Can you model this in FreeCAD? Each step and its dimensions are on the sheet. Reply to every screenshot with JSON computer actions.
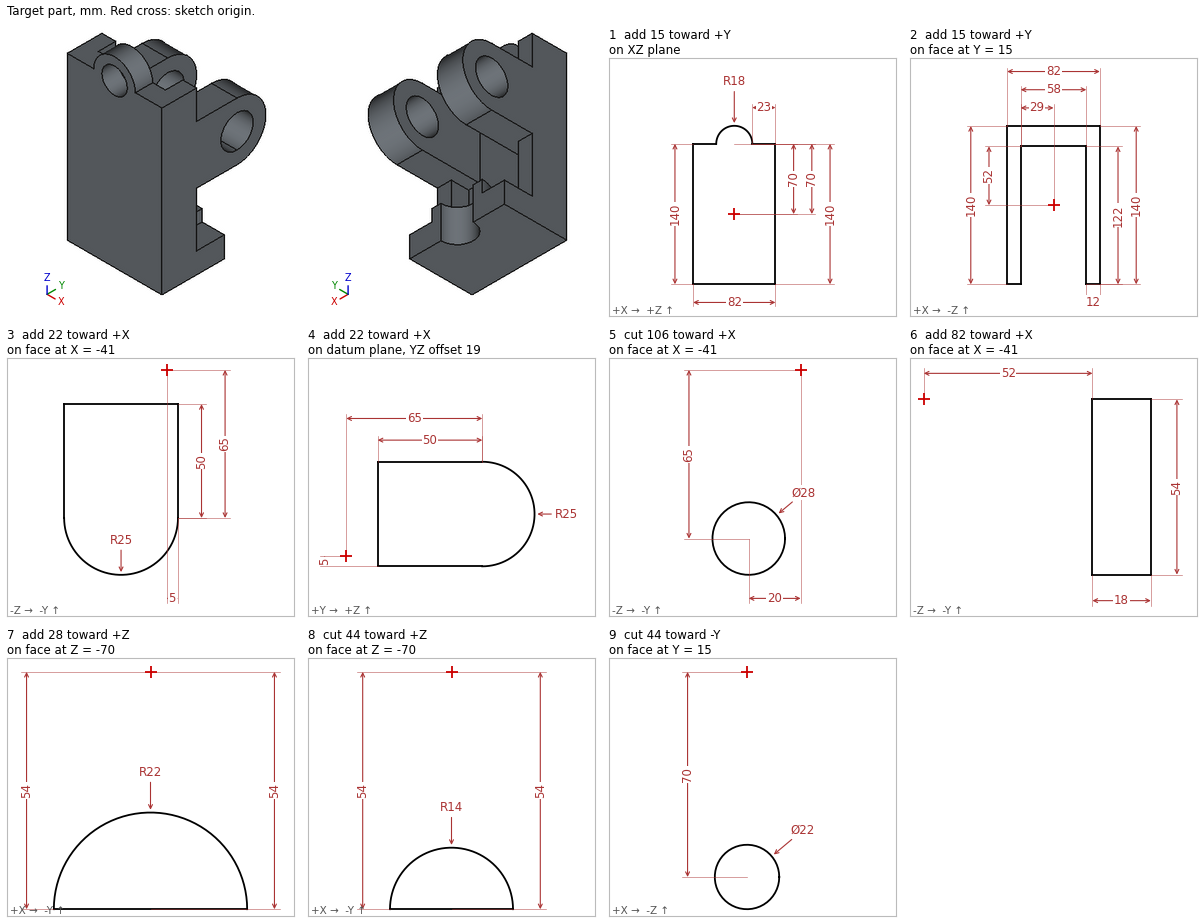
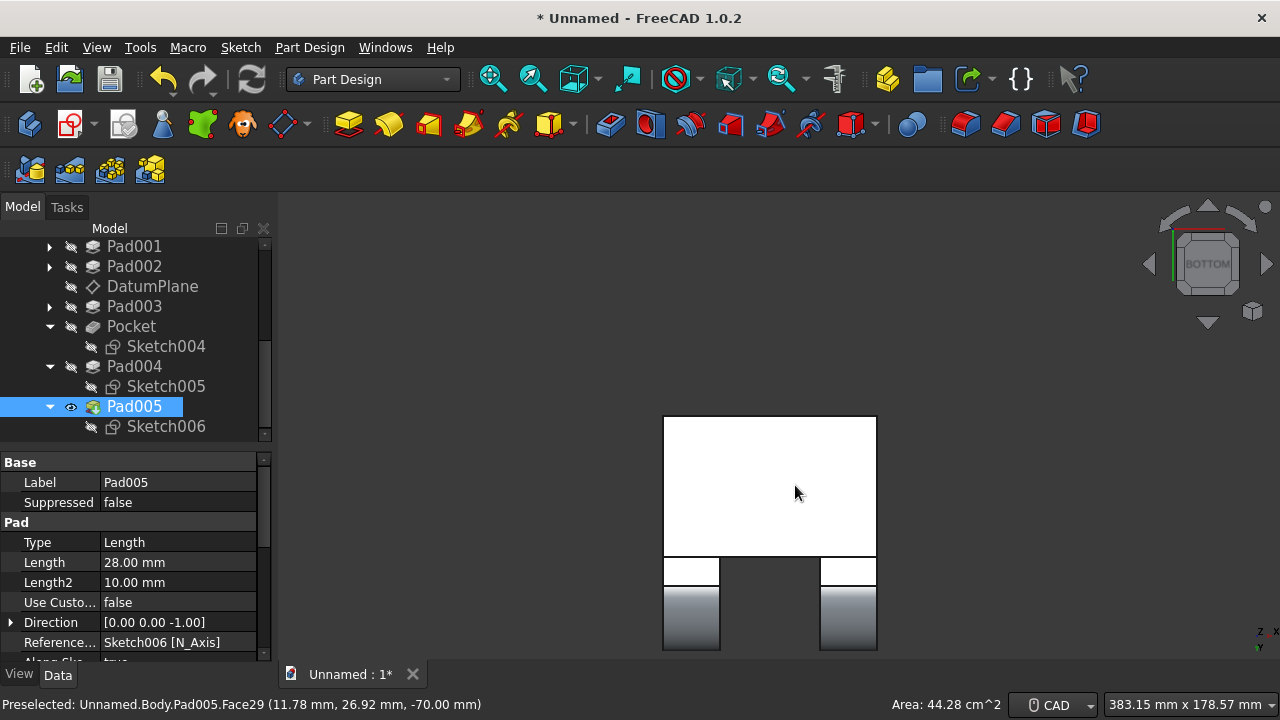
{"action": "left_click", "coordinate": [70, 124]}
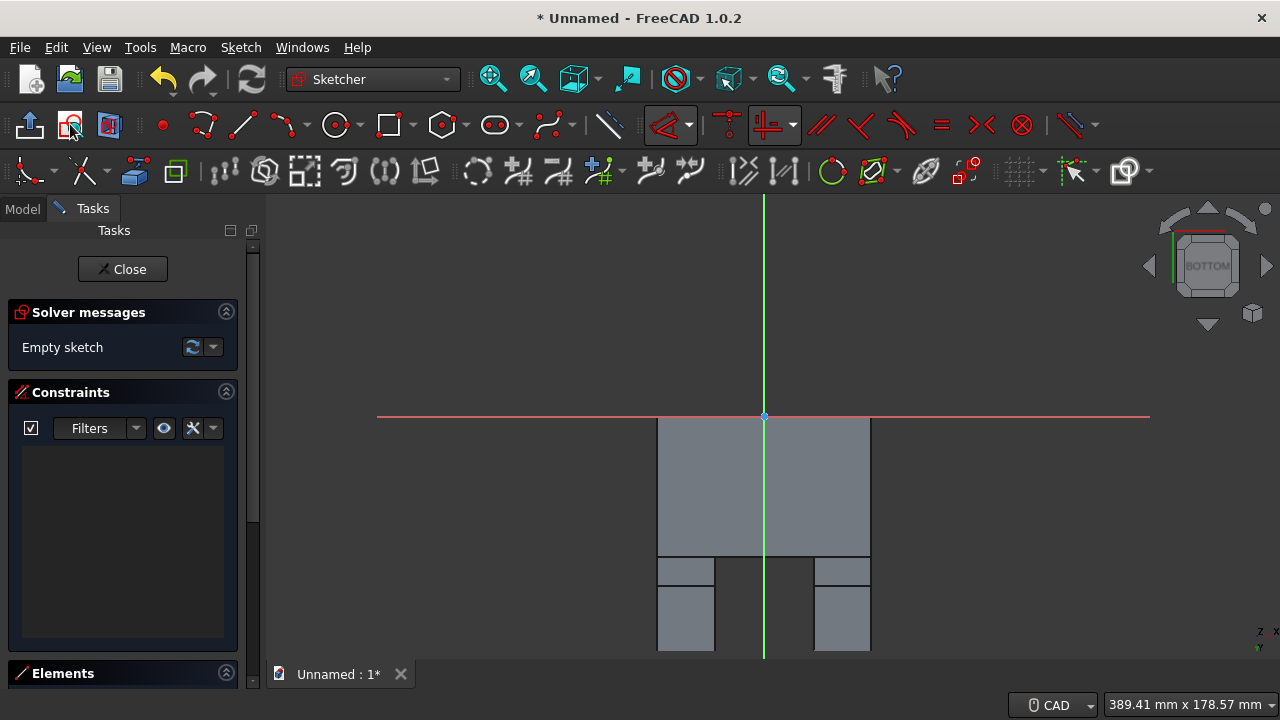
{"action": "scroll", "coordinate": [813, 536], "scroll_direction": "up", "scroll_amount": 4}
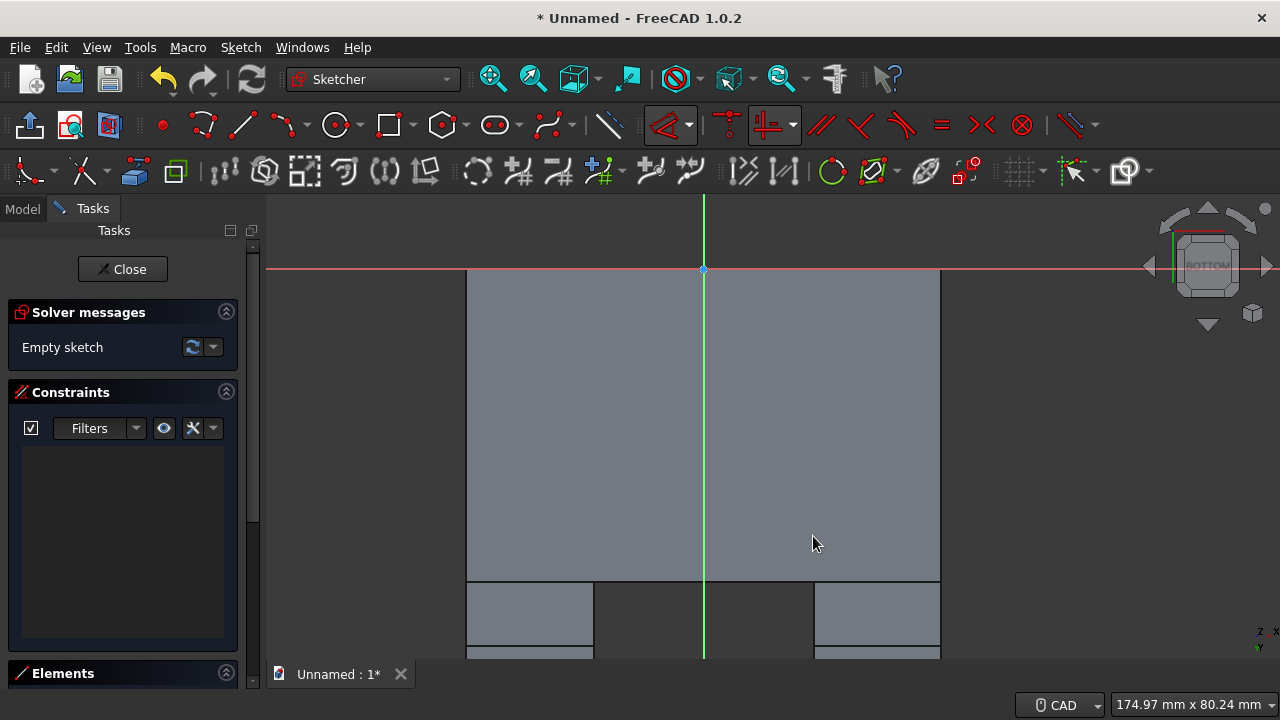
{"action": "key", "text": "g l"}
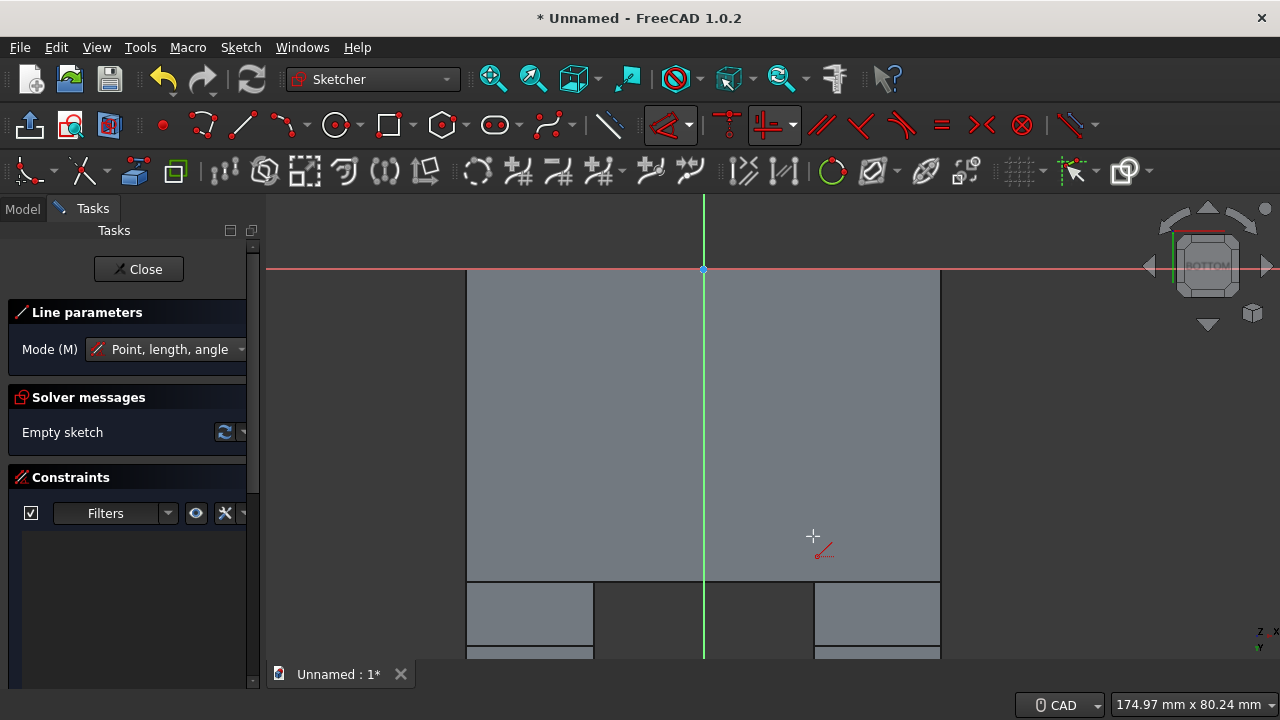
{"action": "left_click", "coordinate": [623, 582]}
{"action": "left_click", "coordinate": [785, 582]}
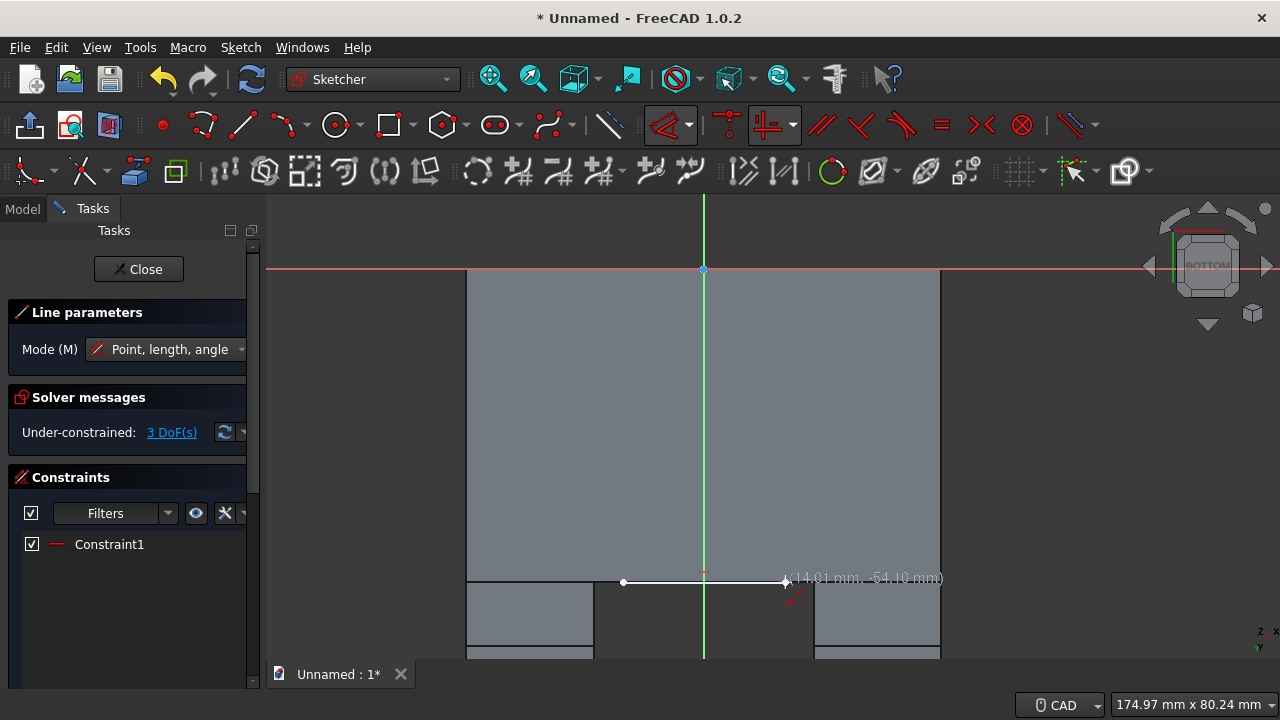
{"action": "key", "text": "g 3 a"}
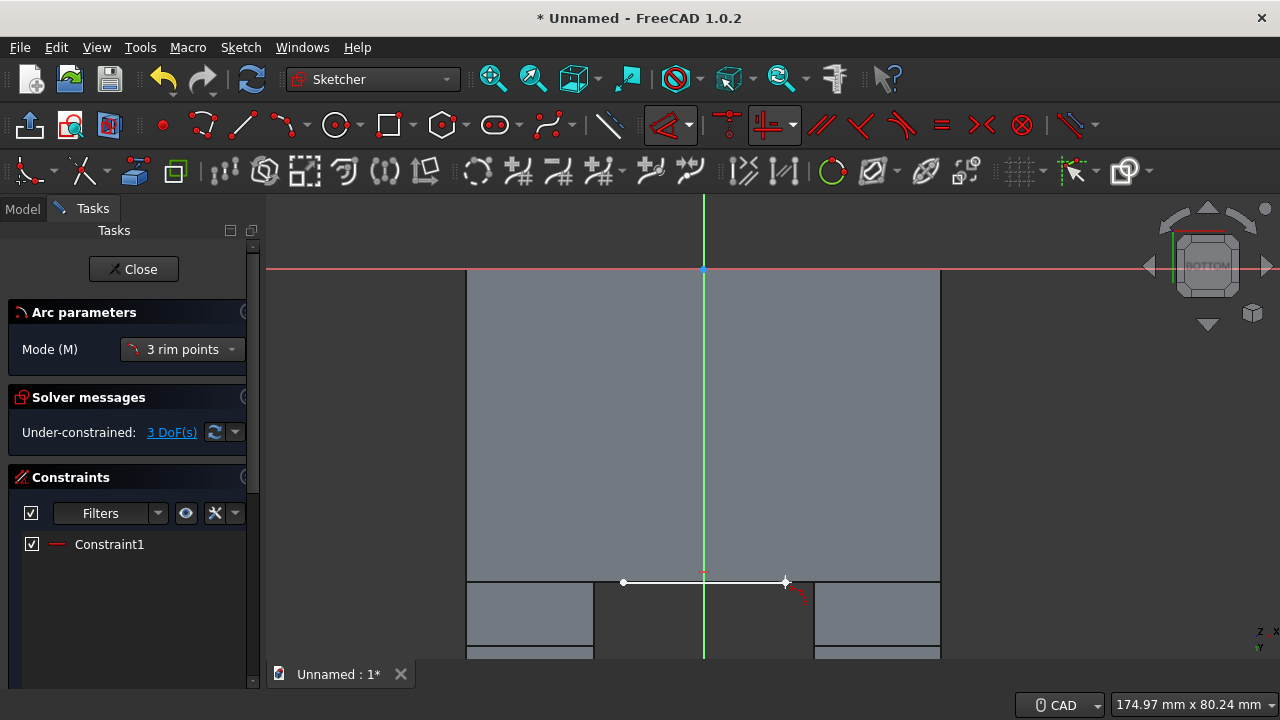
{"action": "left_click", "coordinate": [785, 583]}
{"action": "left_click", "coordinate": [623, 583]}
{"action": "left_click", "coordinate": [729, 505]}
{"action": "key", "text": "Escape"}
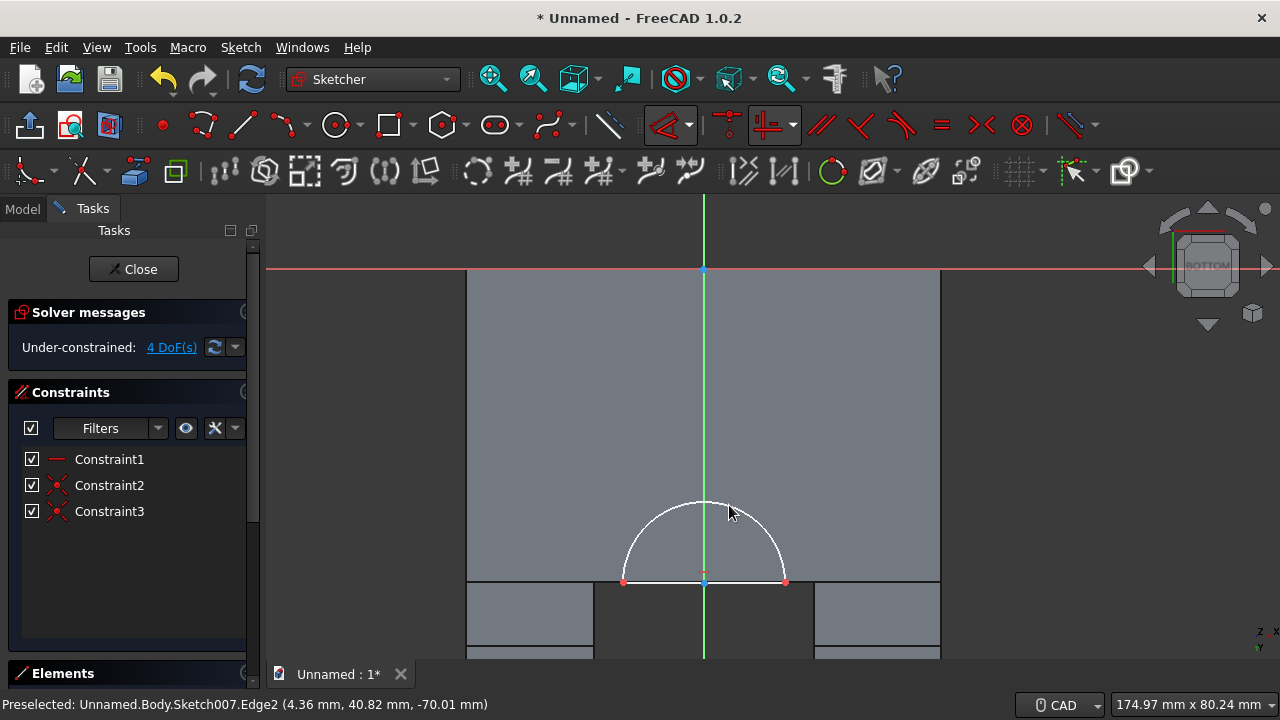
{"action": "left_click", "coordinate": [704, 583]}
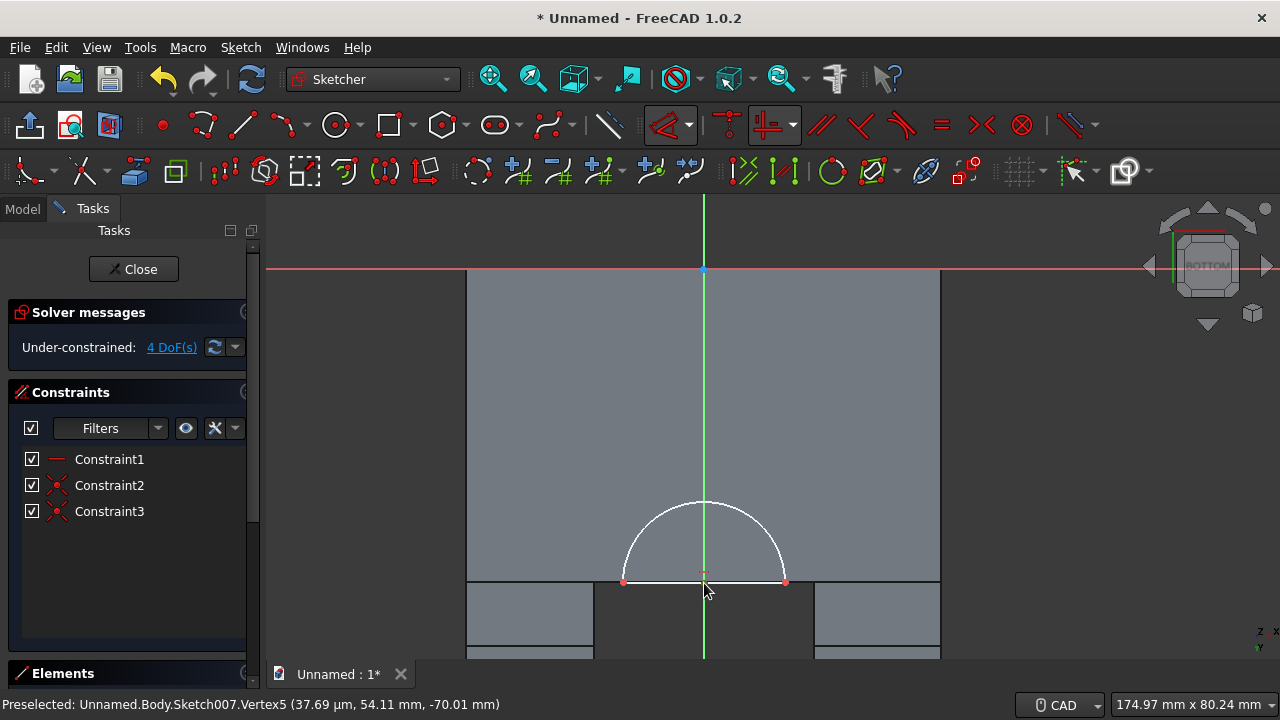
{"action": "left_click", "coordinate": [704, 543]}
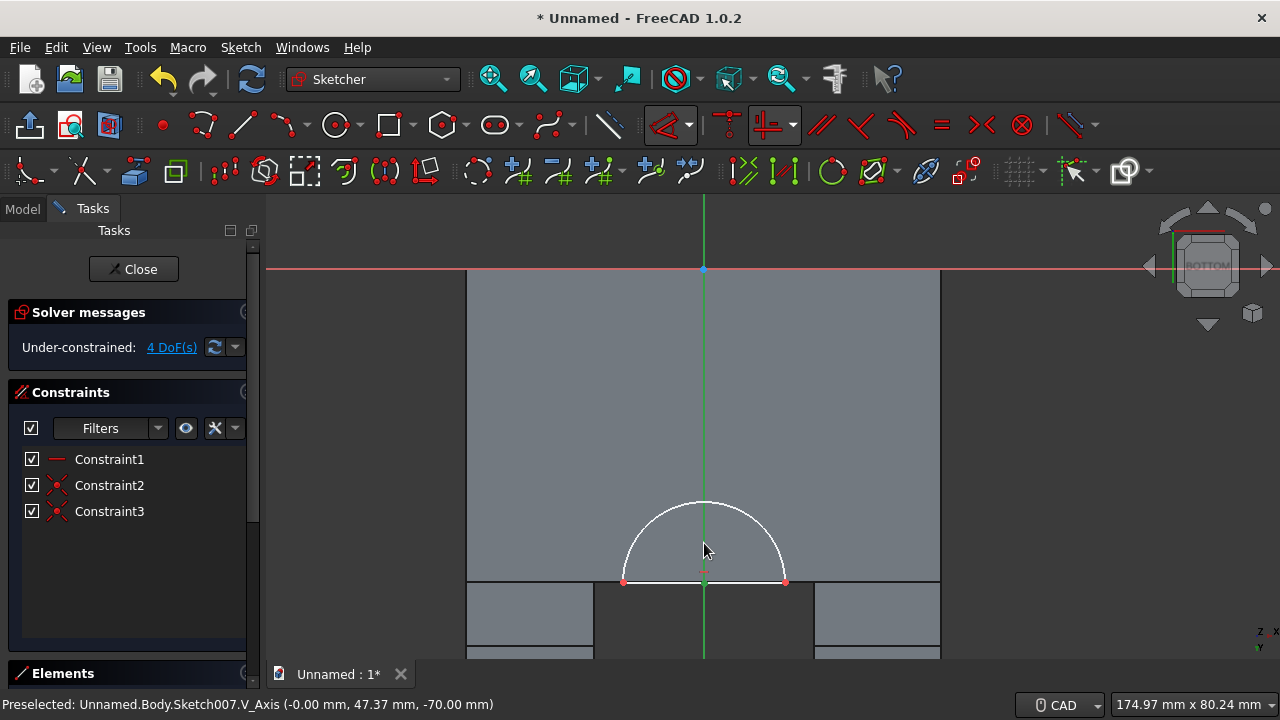
{"action": "key", "text": "c"}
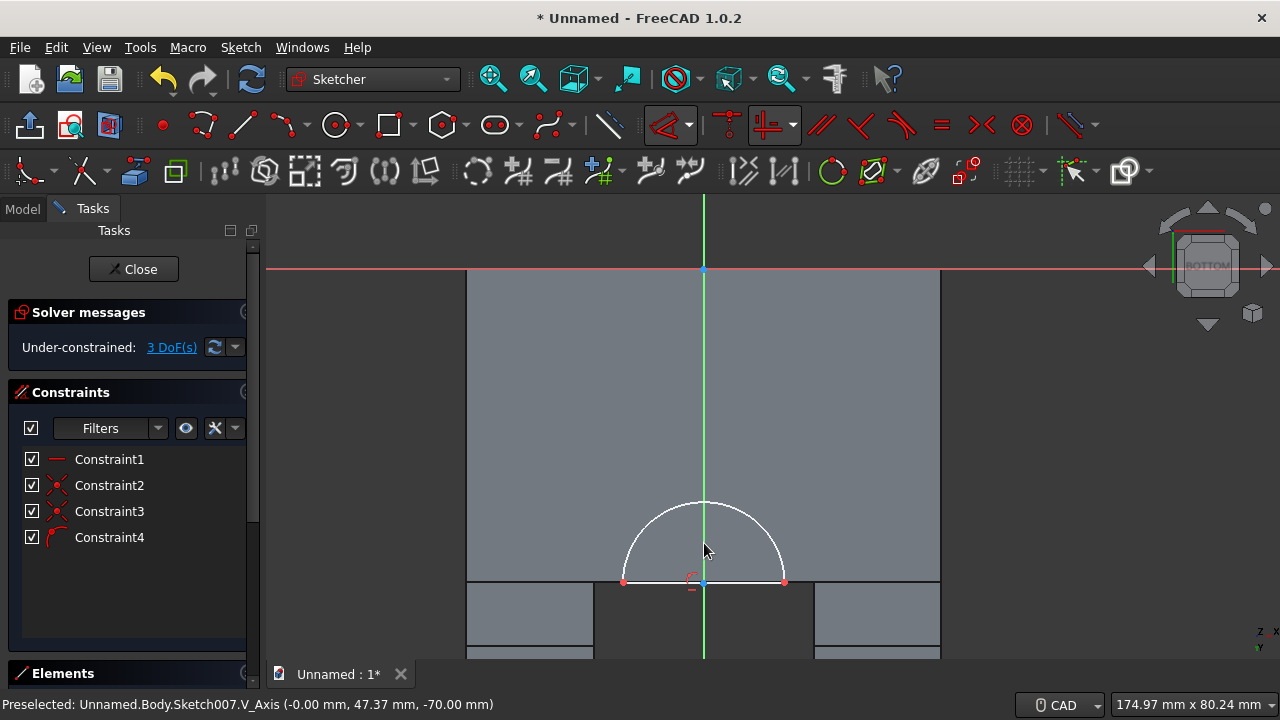
{"action": "left_click", "coordinate": [751, 518]}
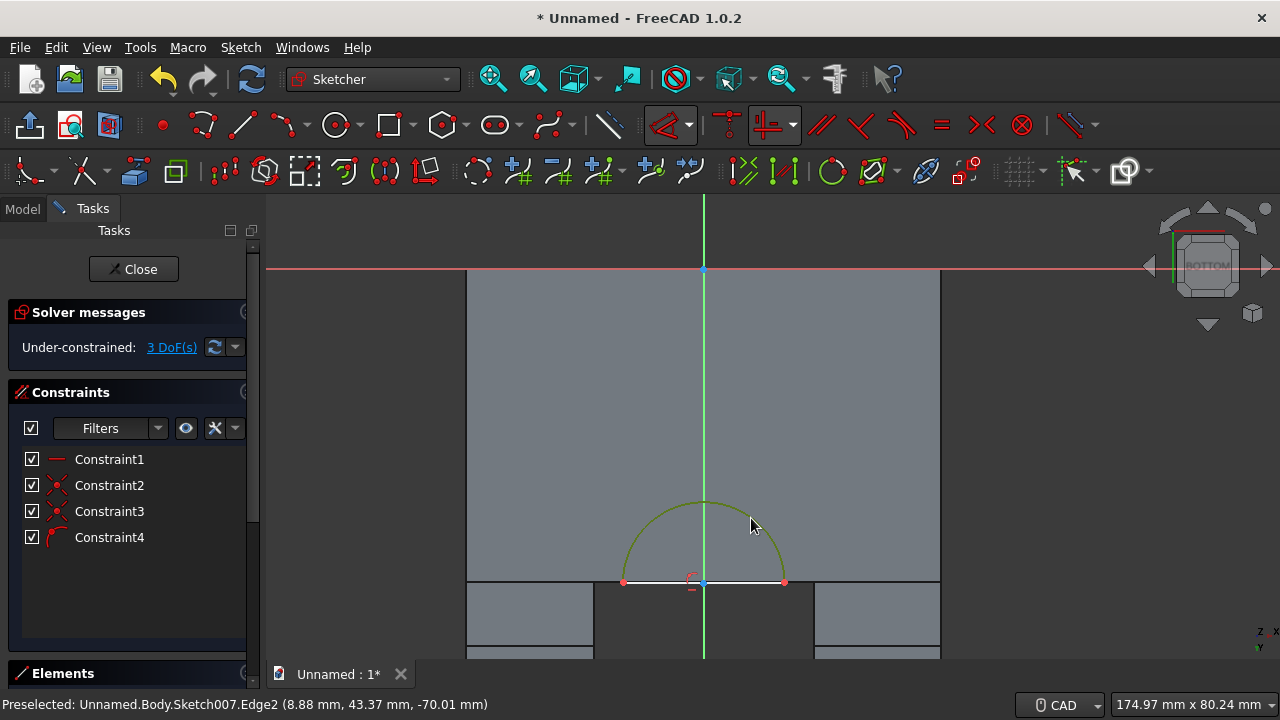
{"action": "key", "text": "k r"}